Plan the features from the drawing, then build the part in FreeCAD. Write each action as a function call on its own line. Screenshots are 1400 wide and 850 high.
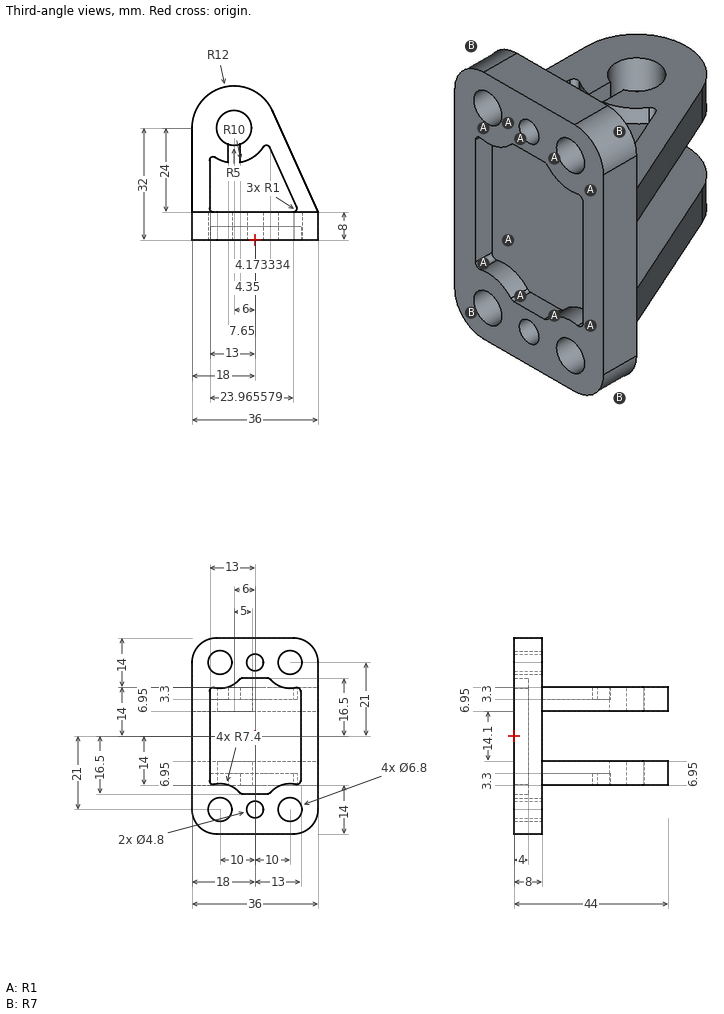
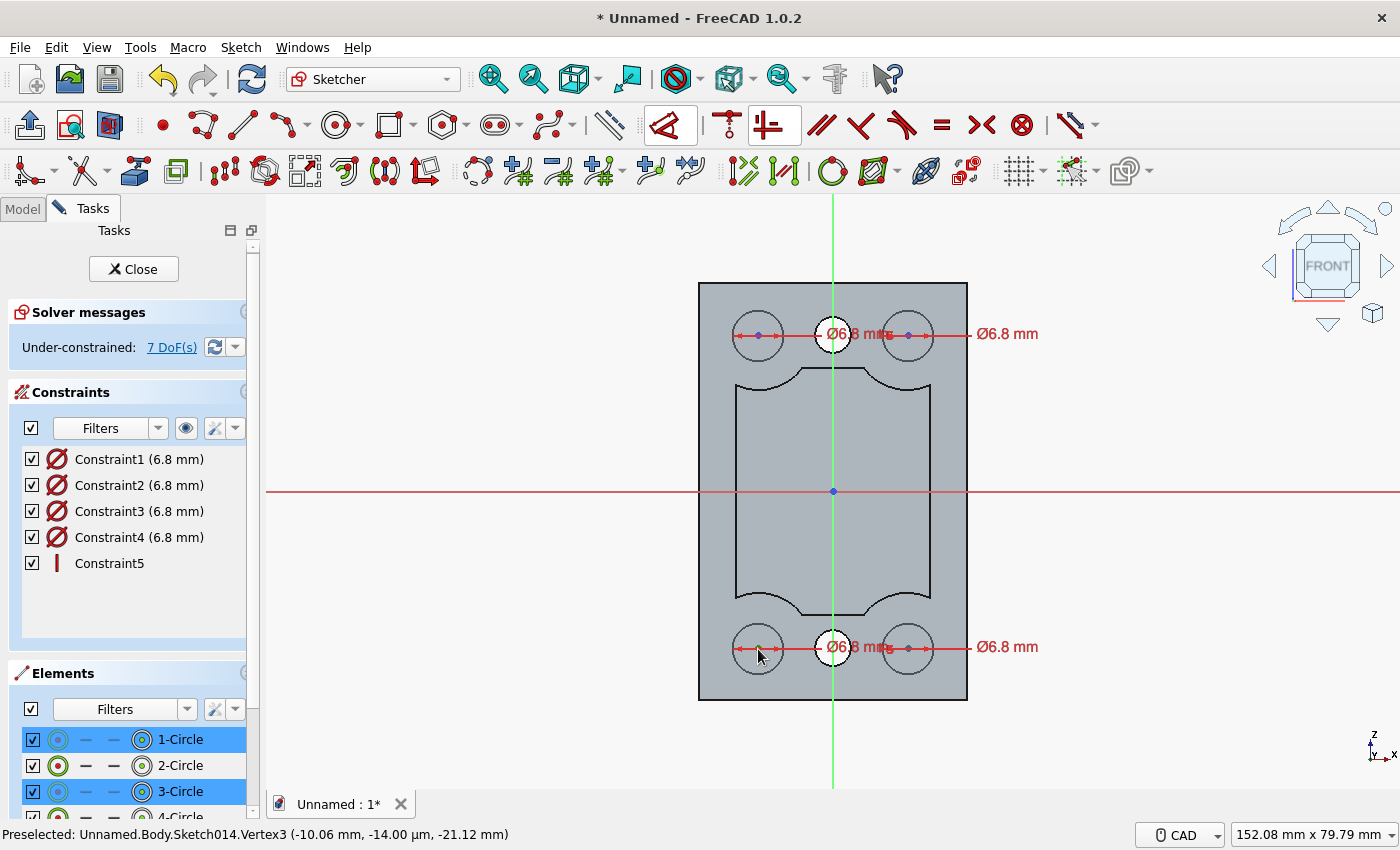
key(h)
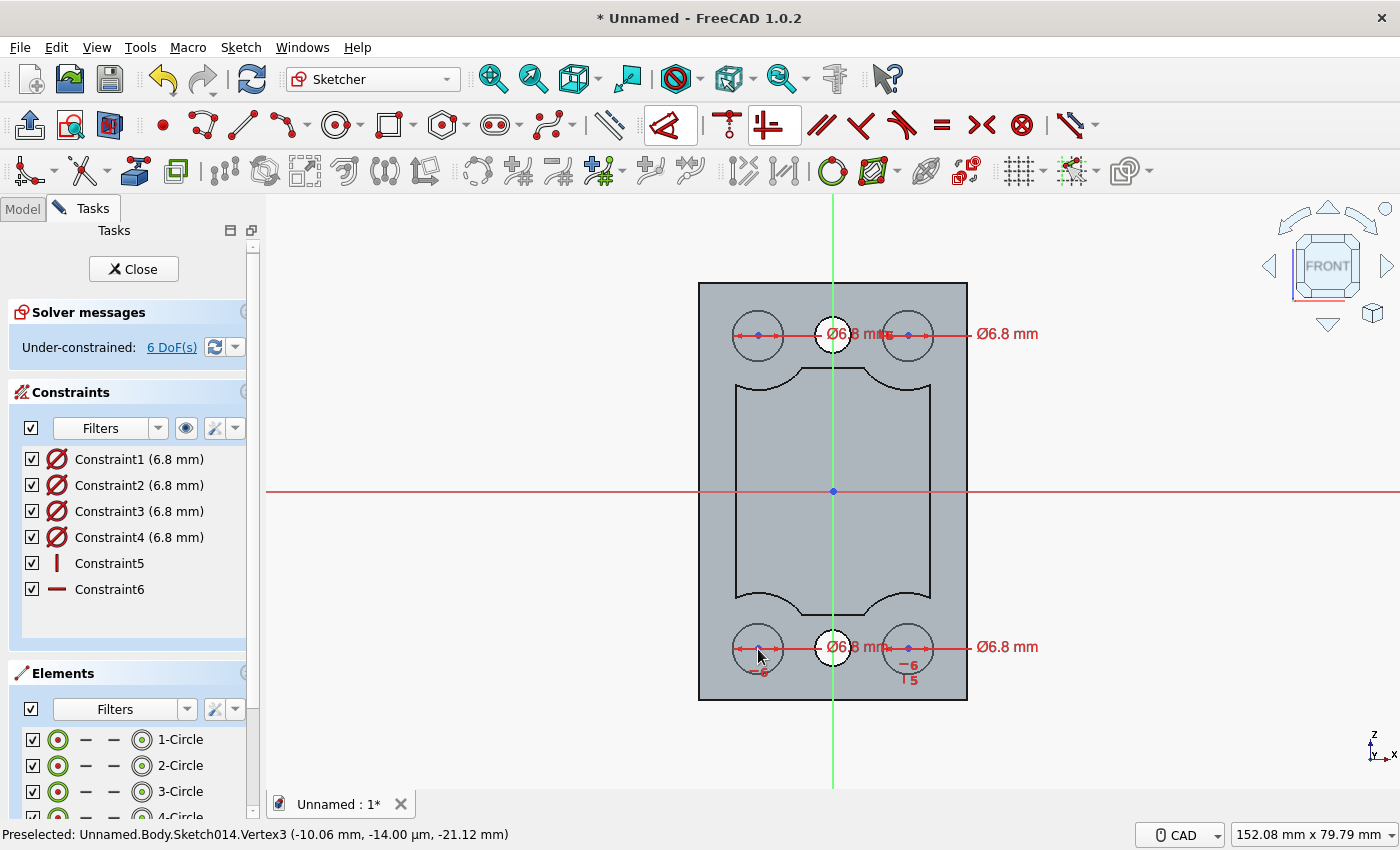
click(758, 649)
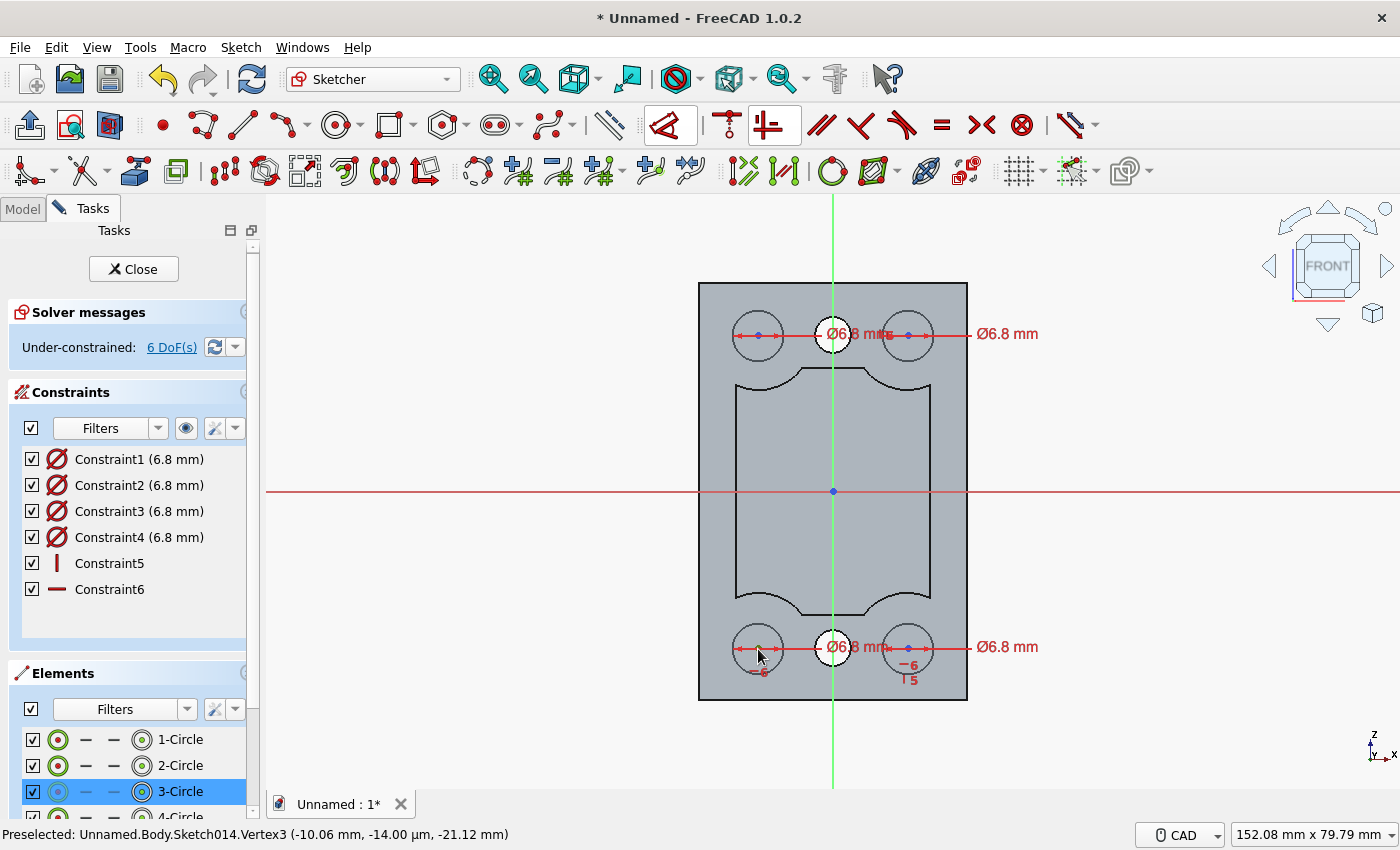
click(758, 336)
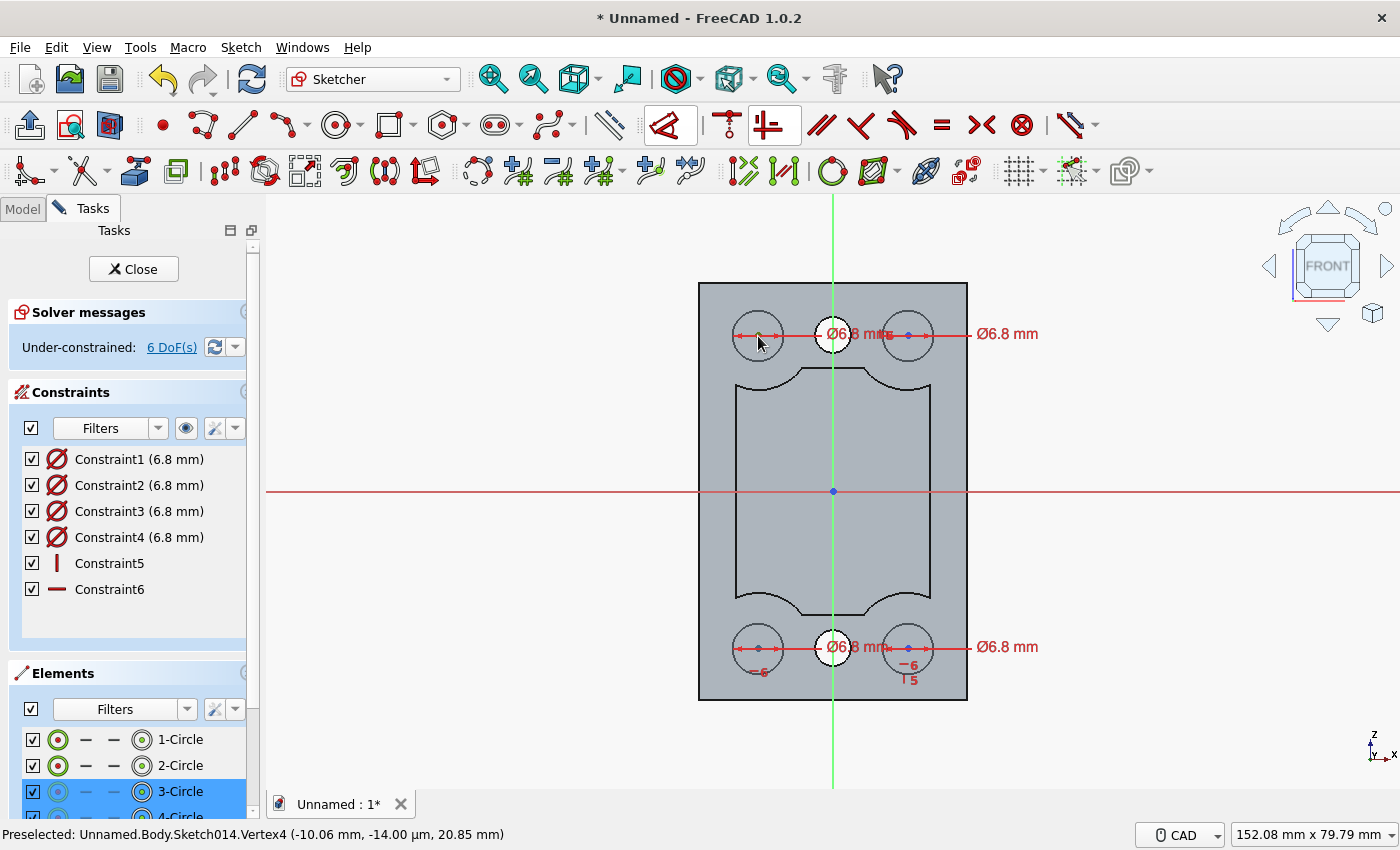
key(v)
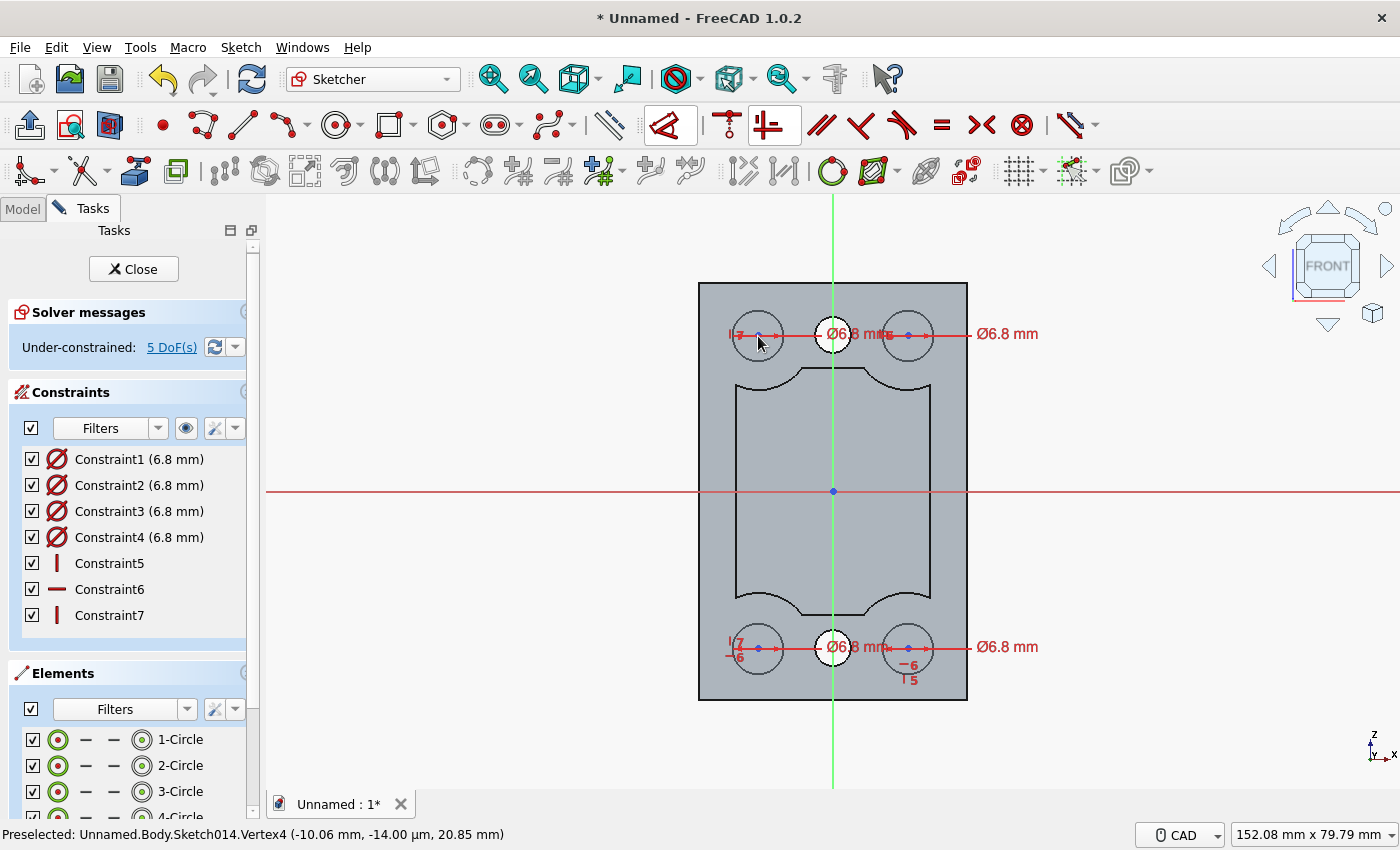
click(908, 336)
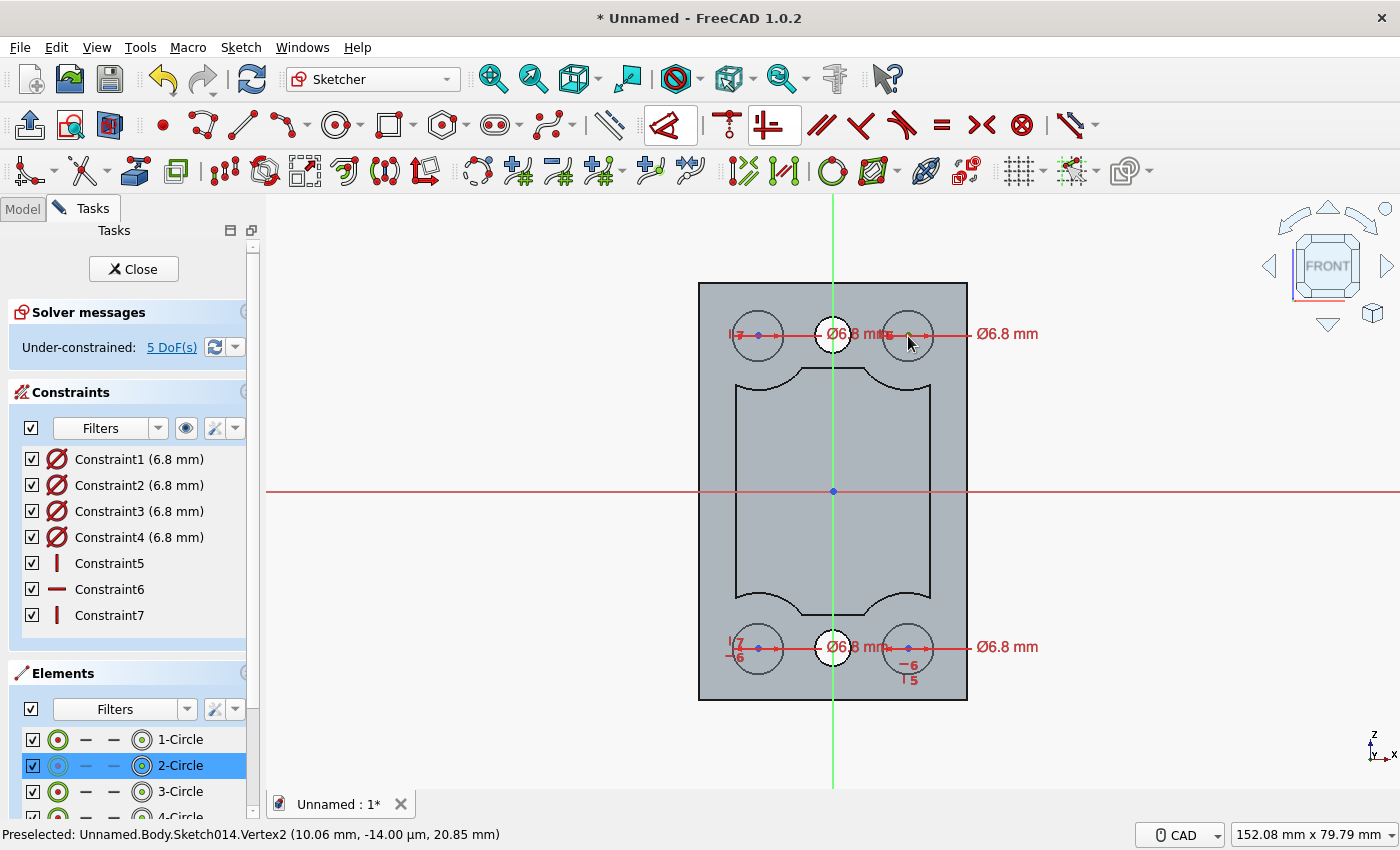
click(758, 336)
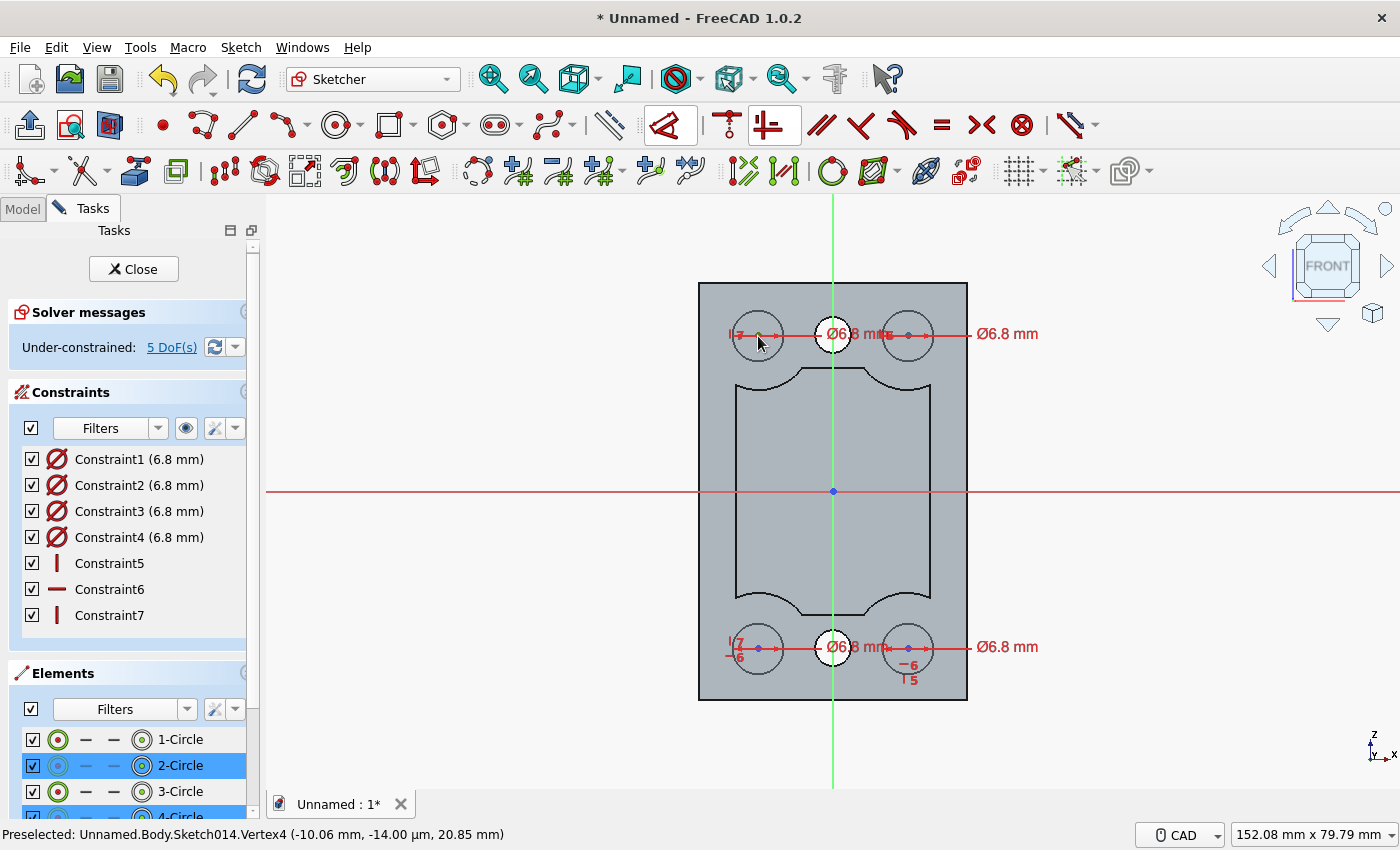
key(h)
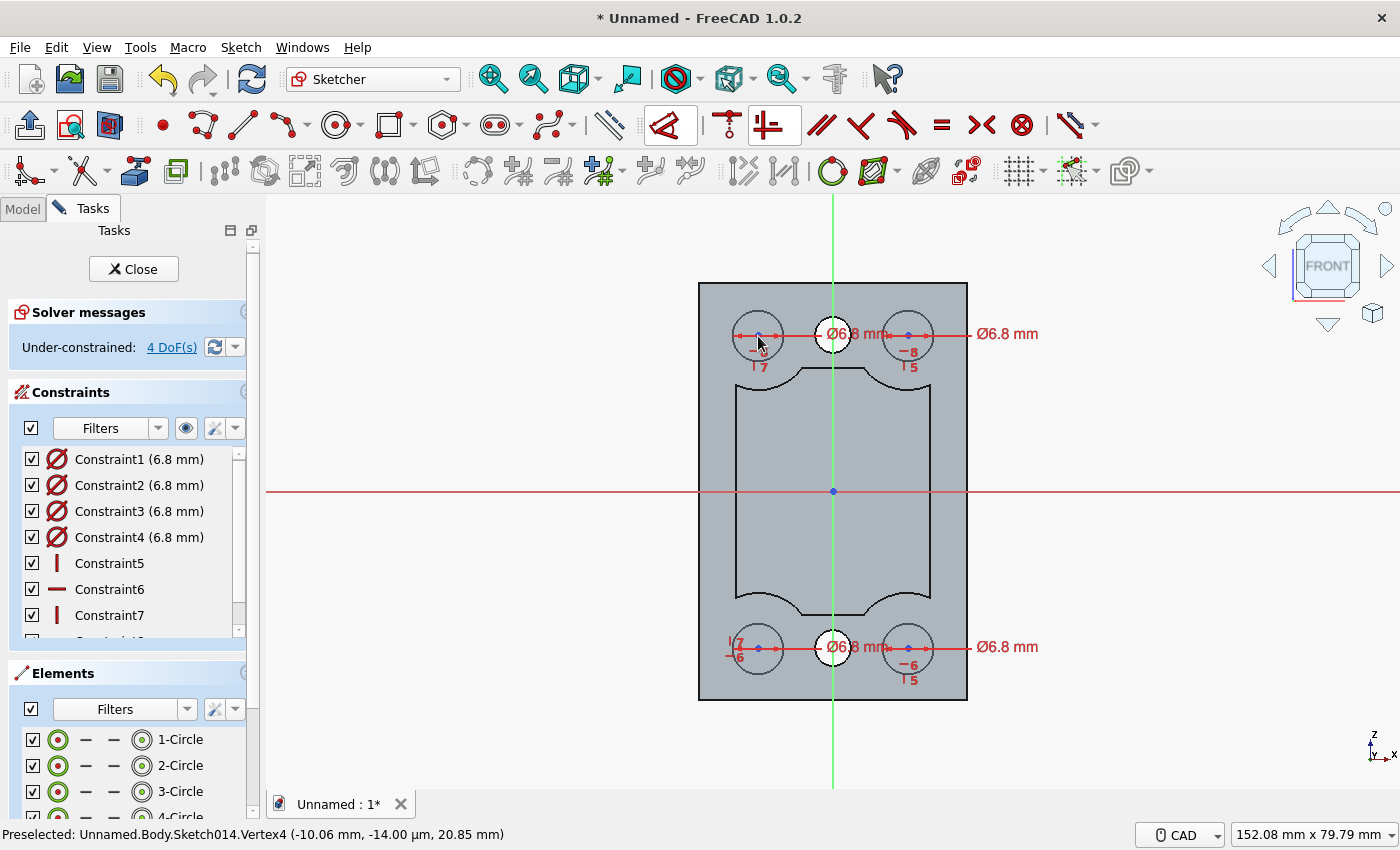
click(908, 649)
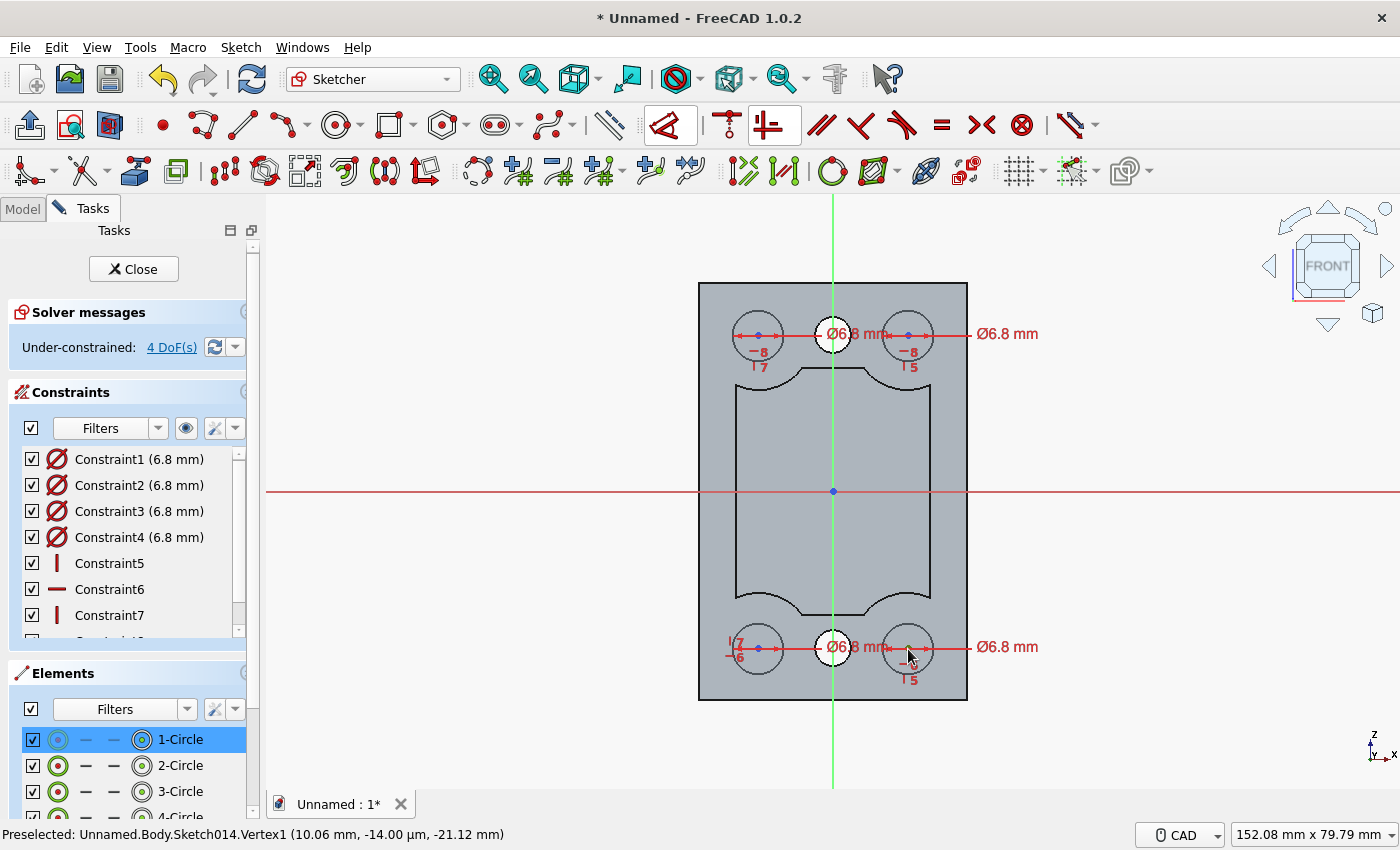
click(692, 126)